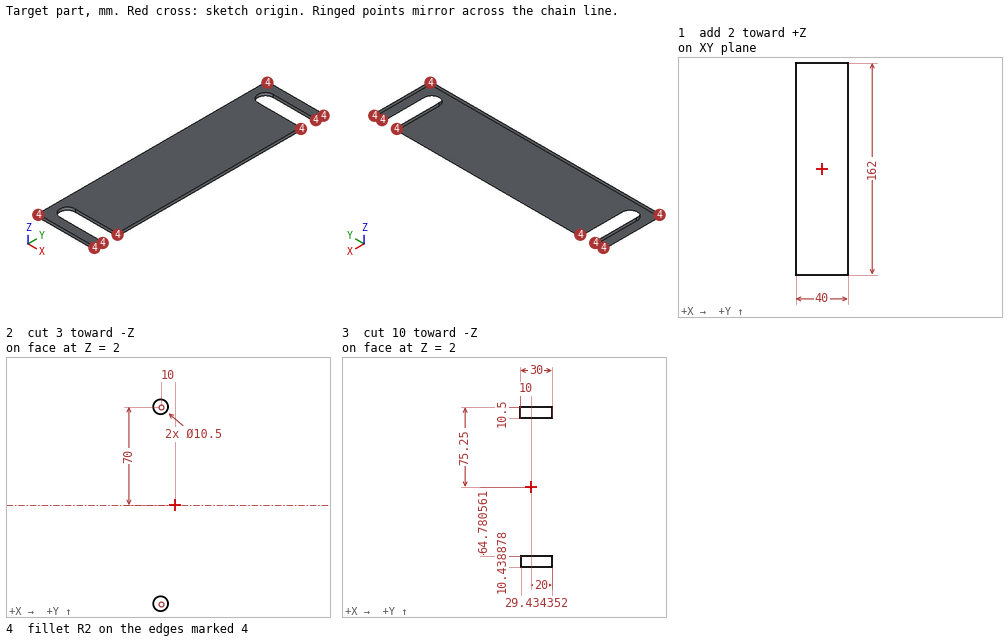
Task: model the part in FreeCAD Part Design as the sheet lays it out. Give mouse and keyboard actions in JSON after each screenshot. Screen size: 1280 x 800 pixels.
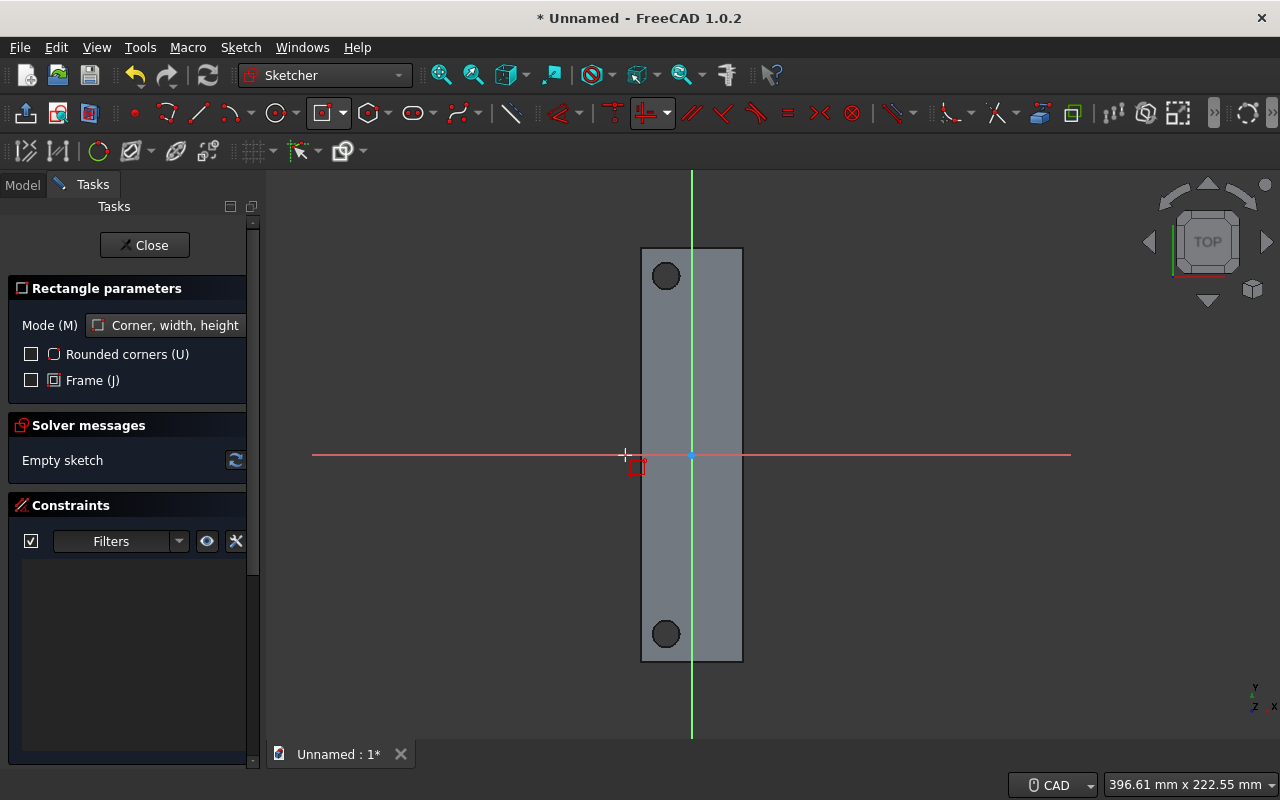
{"action": "left_click", "coordinate": [666, 263]}
{"action": "left_click", "coordinate": [743, 290]}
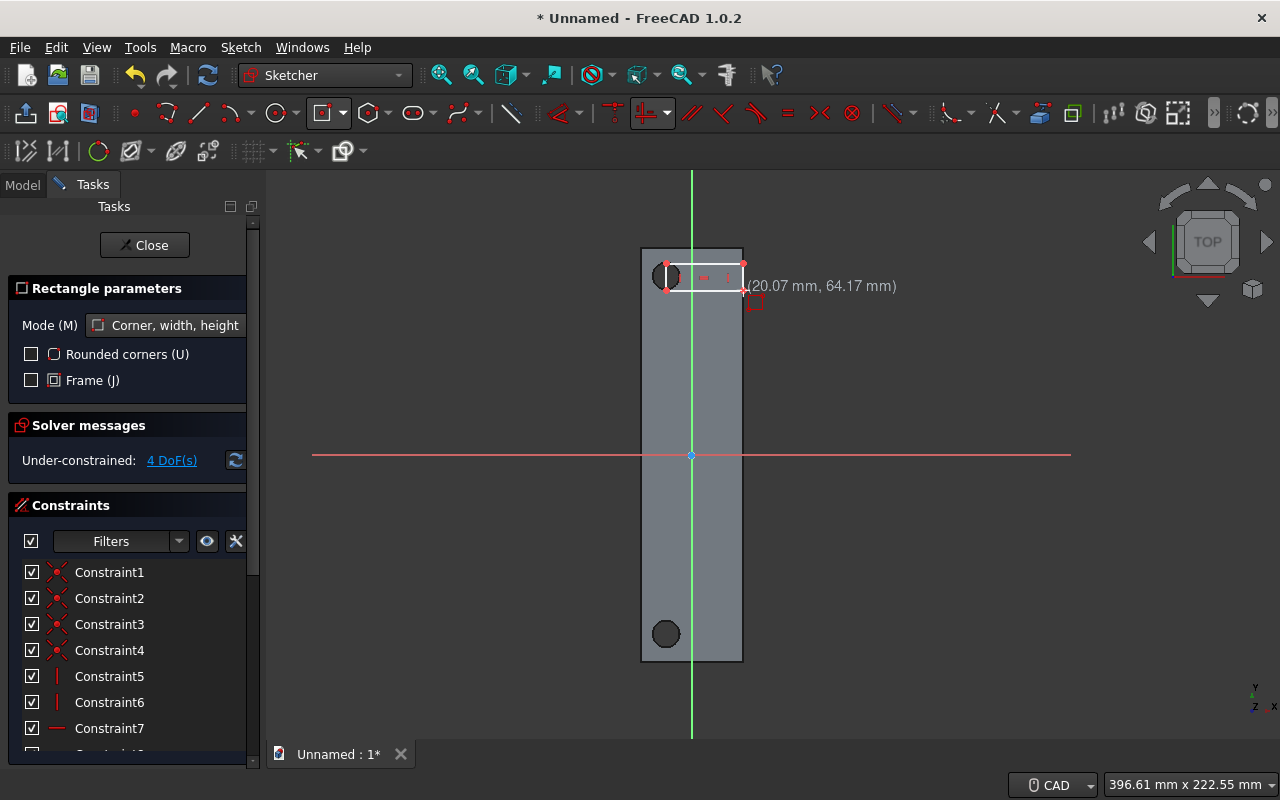
{"action": "left_click", "coordinate": [668, 621]}
{"action": "left_click", "coordinate": [743, 647]}
{"action": "key", "text": "Escape"}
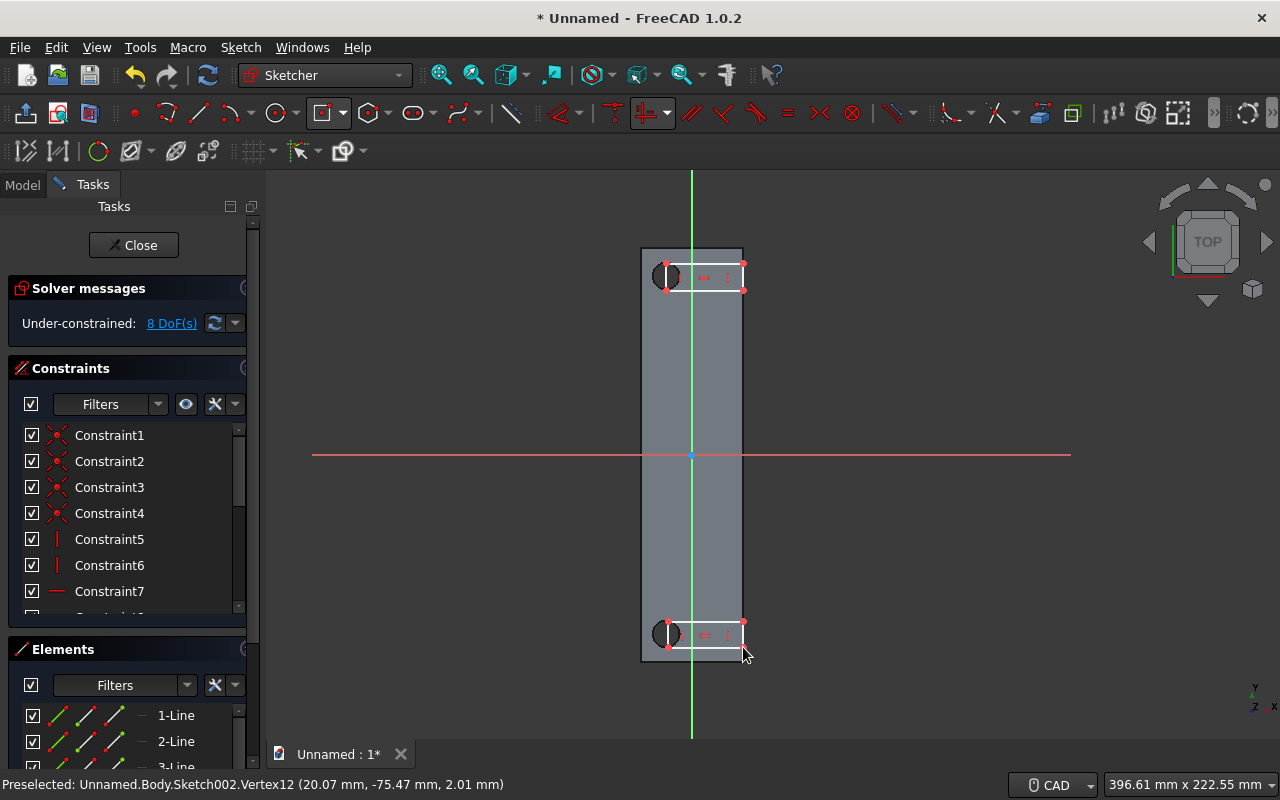
{"action": "key", "text": "d"}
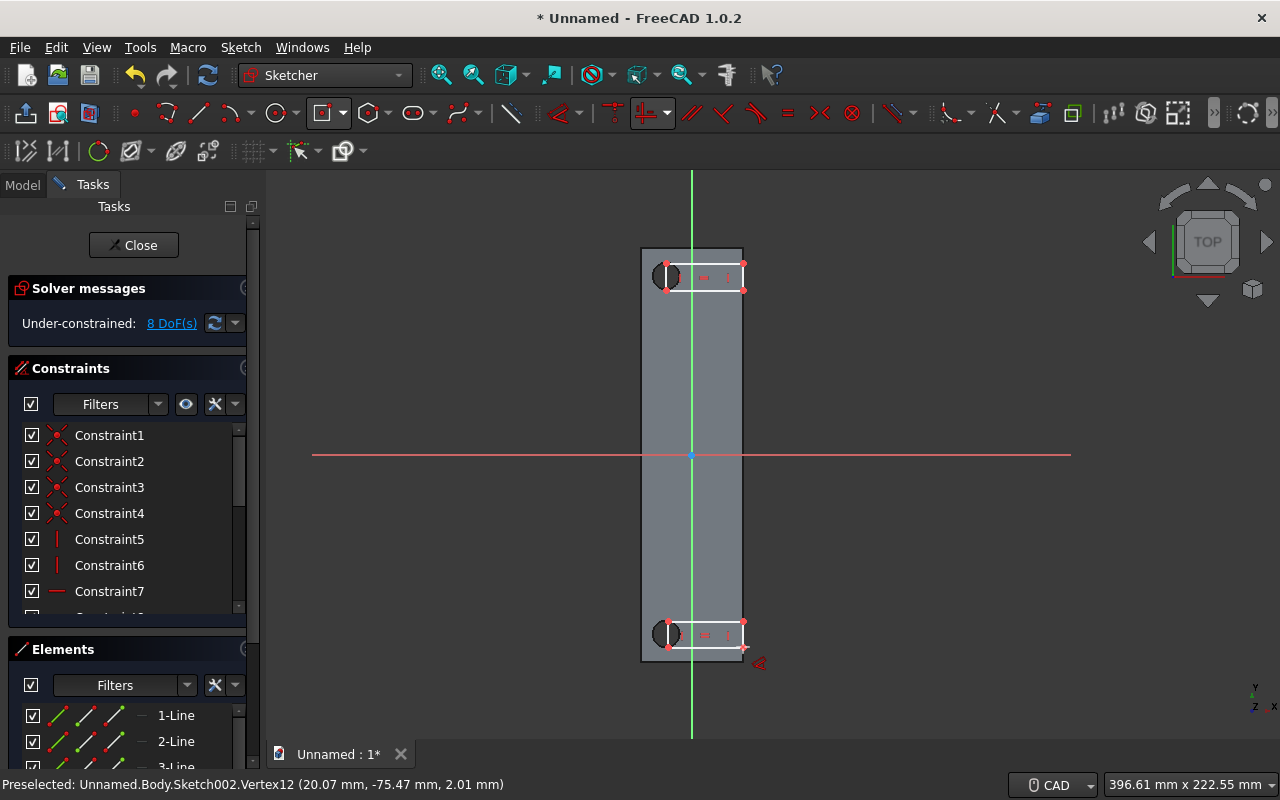
{"action": "left_click", "coordinate": [689, 291]}
{"action": "left_click", "coordinate": [722, 325]}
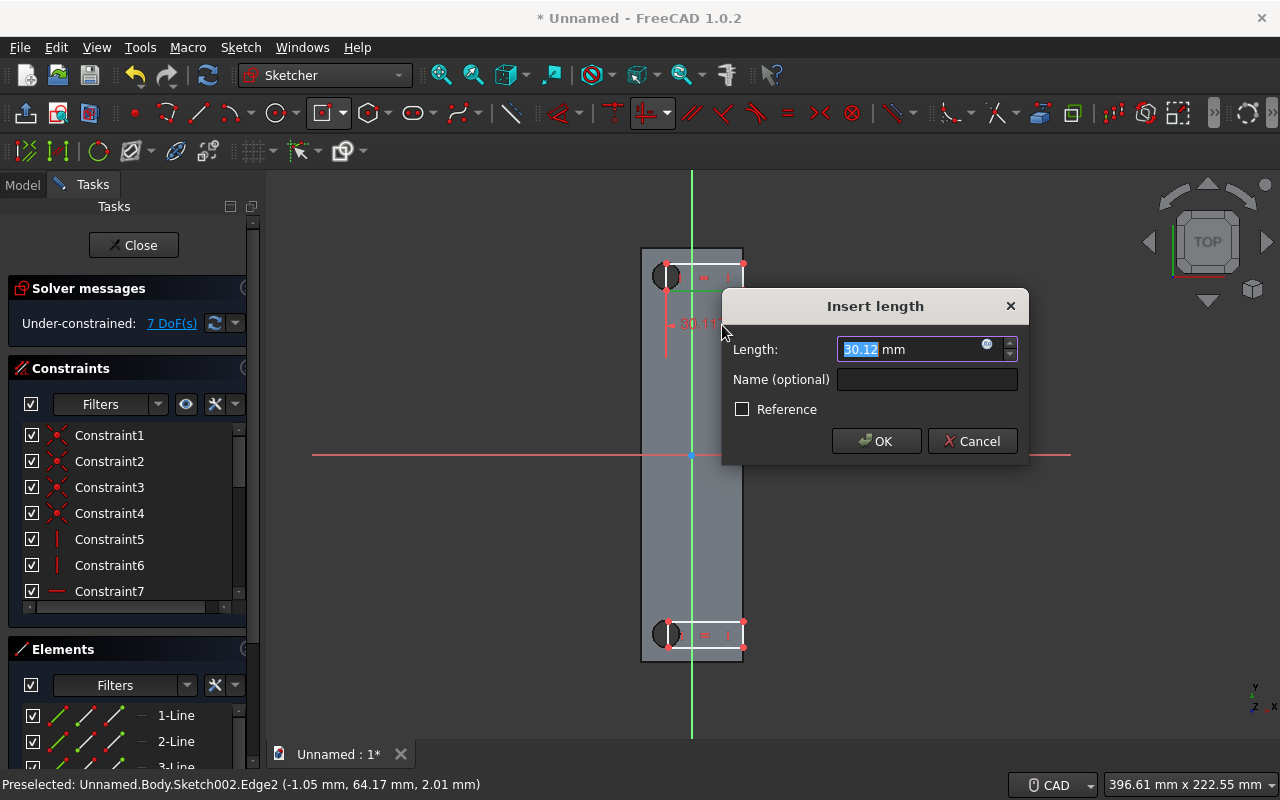
{"action": "type", "text": "30"}
{"action": "key", "text": "Return"}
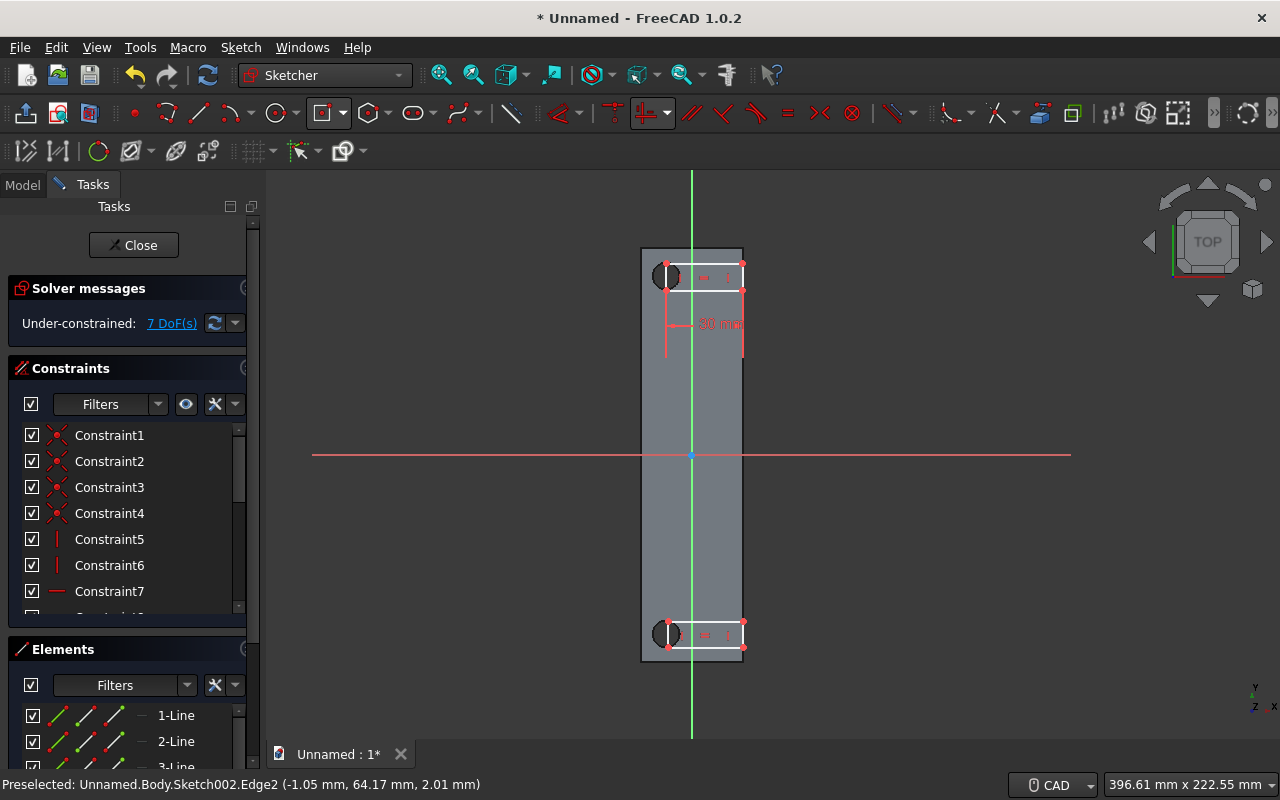
{"action": "scroll", "coordinate": [666, 264], "scroll_direction": "up", "scroll_amount": 3}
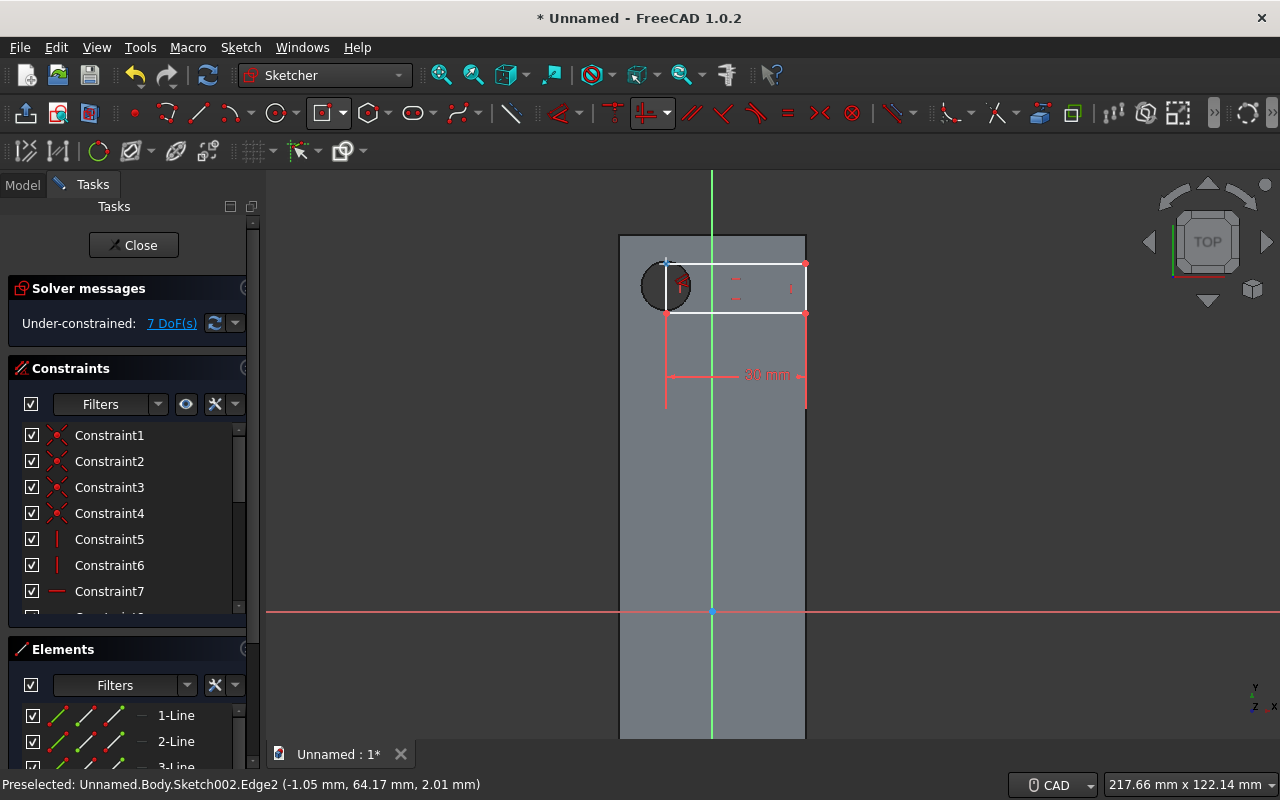
{"action": "left_click", "coordinate": [666, 264]}
{"action": "left_click", "coordinate": [689, 230]}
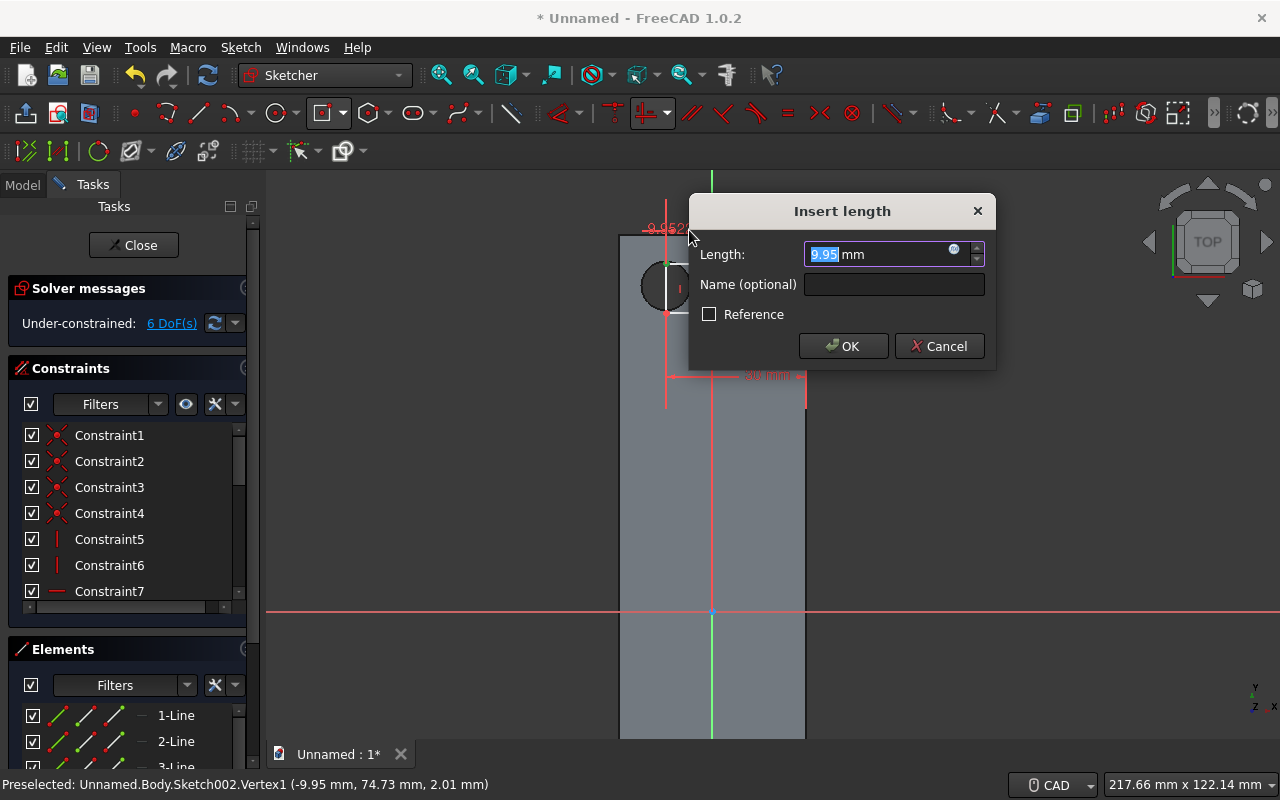
{"action": "type", "text": "10"}
{"action": "key", "text": "Return"}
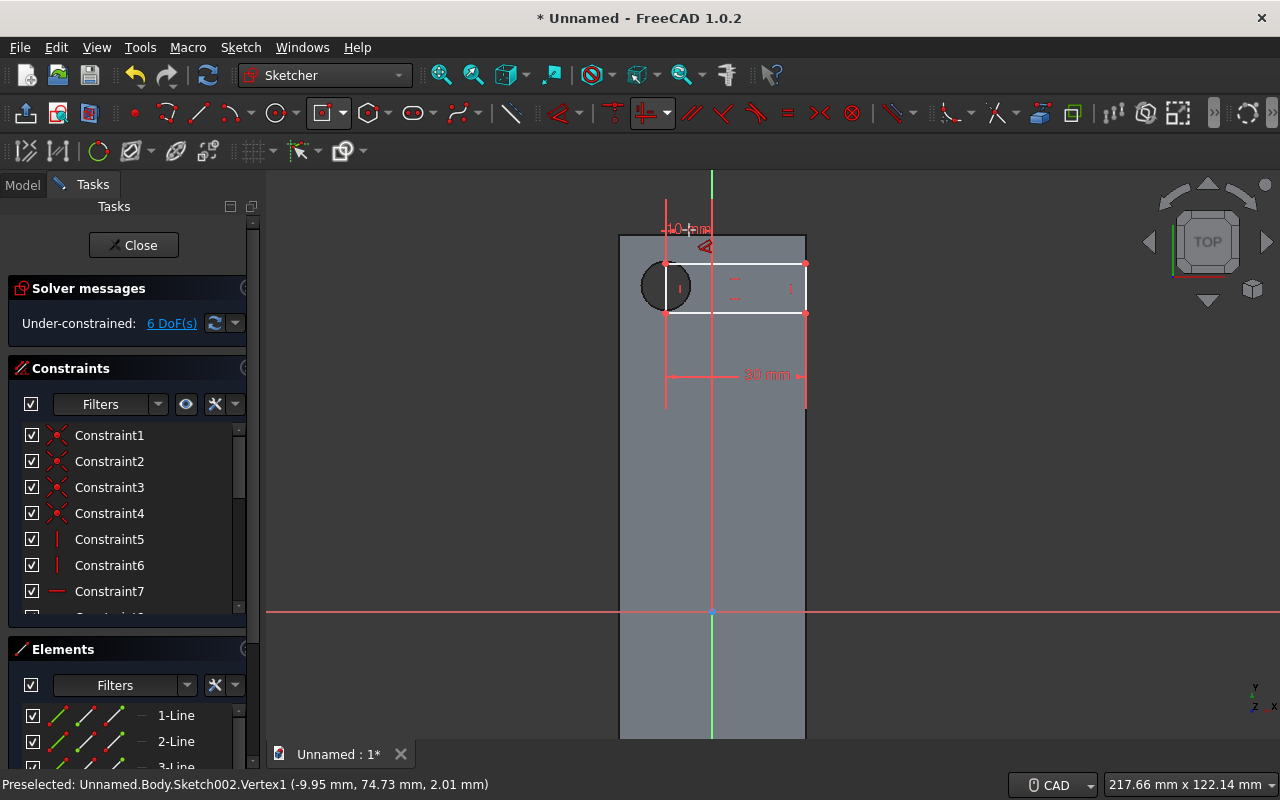
{"action": "scroll", "coordinate": [666, 263], "scroll_direction": "down", "scroll_amount": 3}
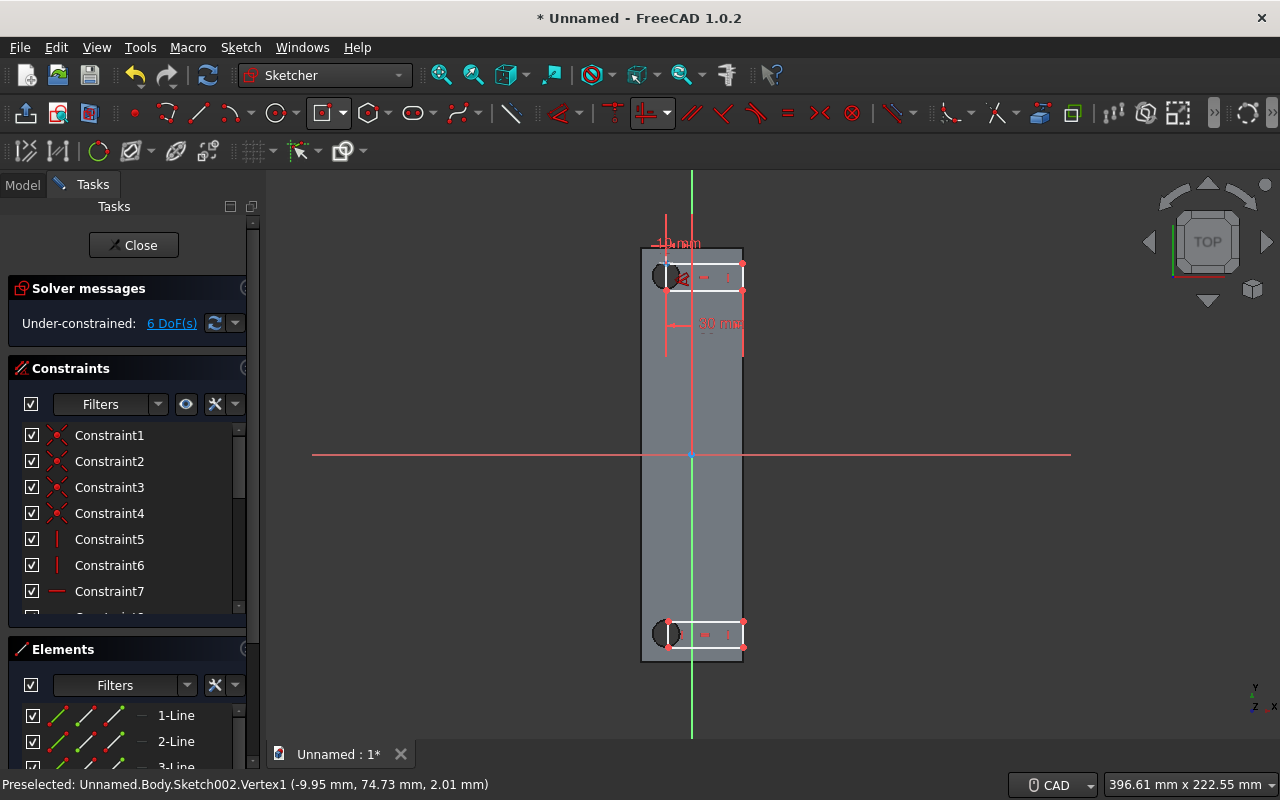
{"action": "left_click", "coordinate": [743, 648]}
{"action": "left_click", "coordinate": [717, 682]}